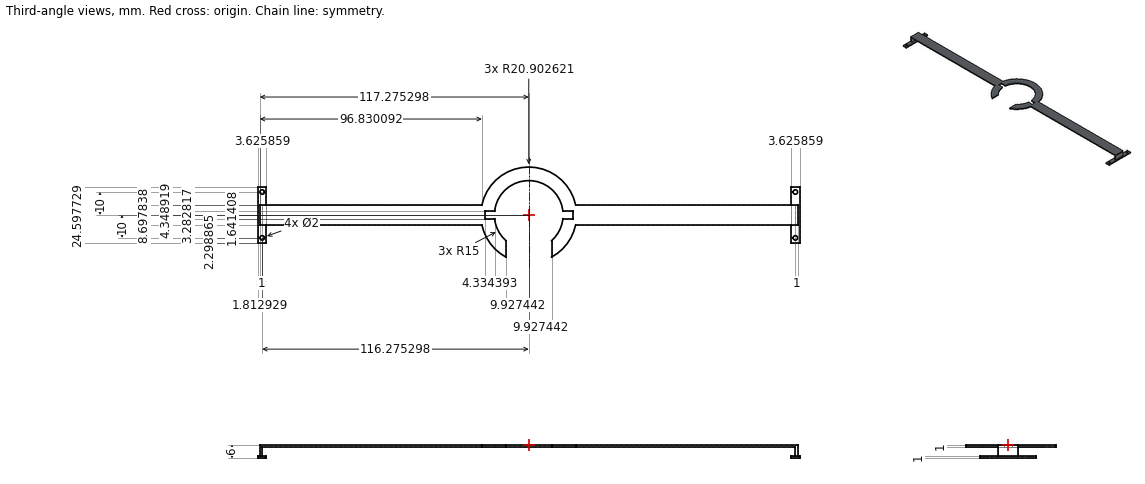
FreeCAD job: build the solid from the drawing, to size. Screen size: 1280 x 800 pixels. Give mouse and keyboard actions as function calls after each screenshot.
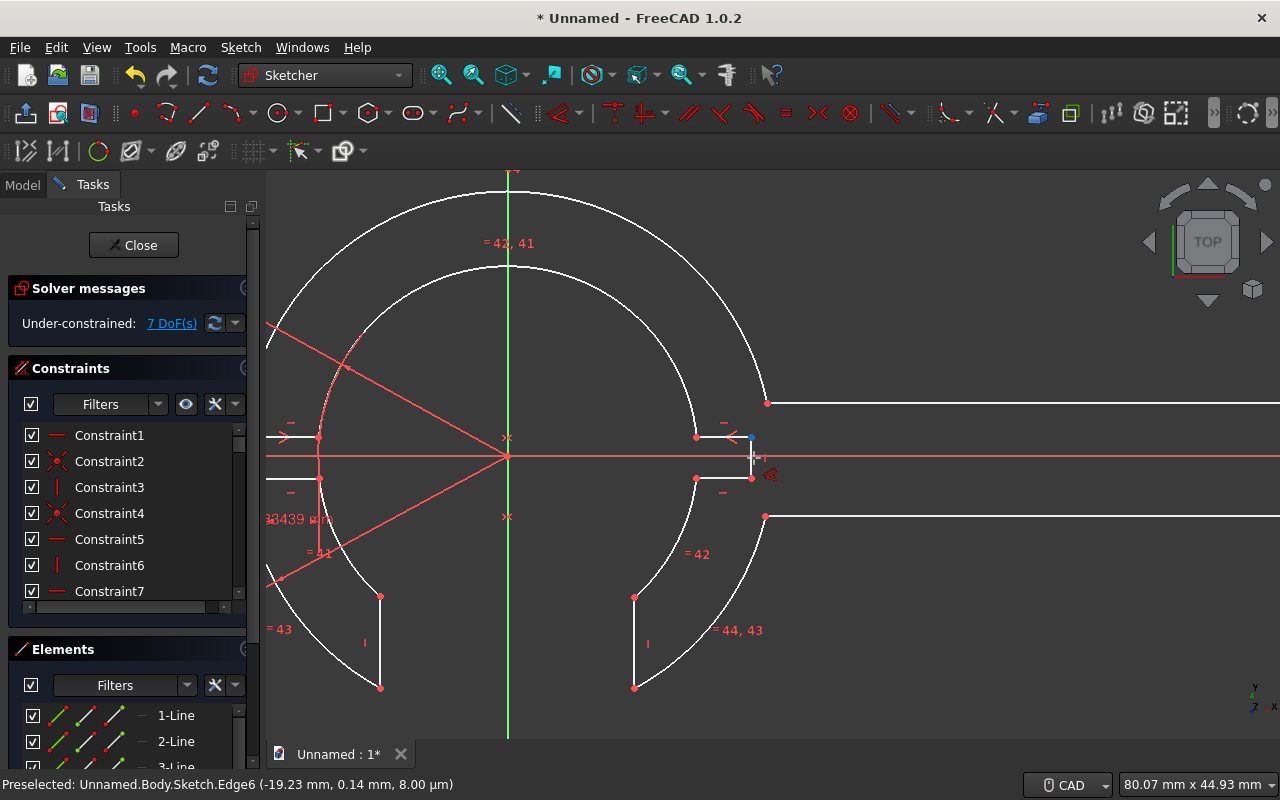
click(751, 454)
click(785, 472)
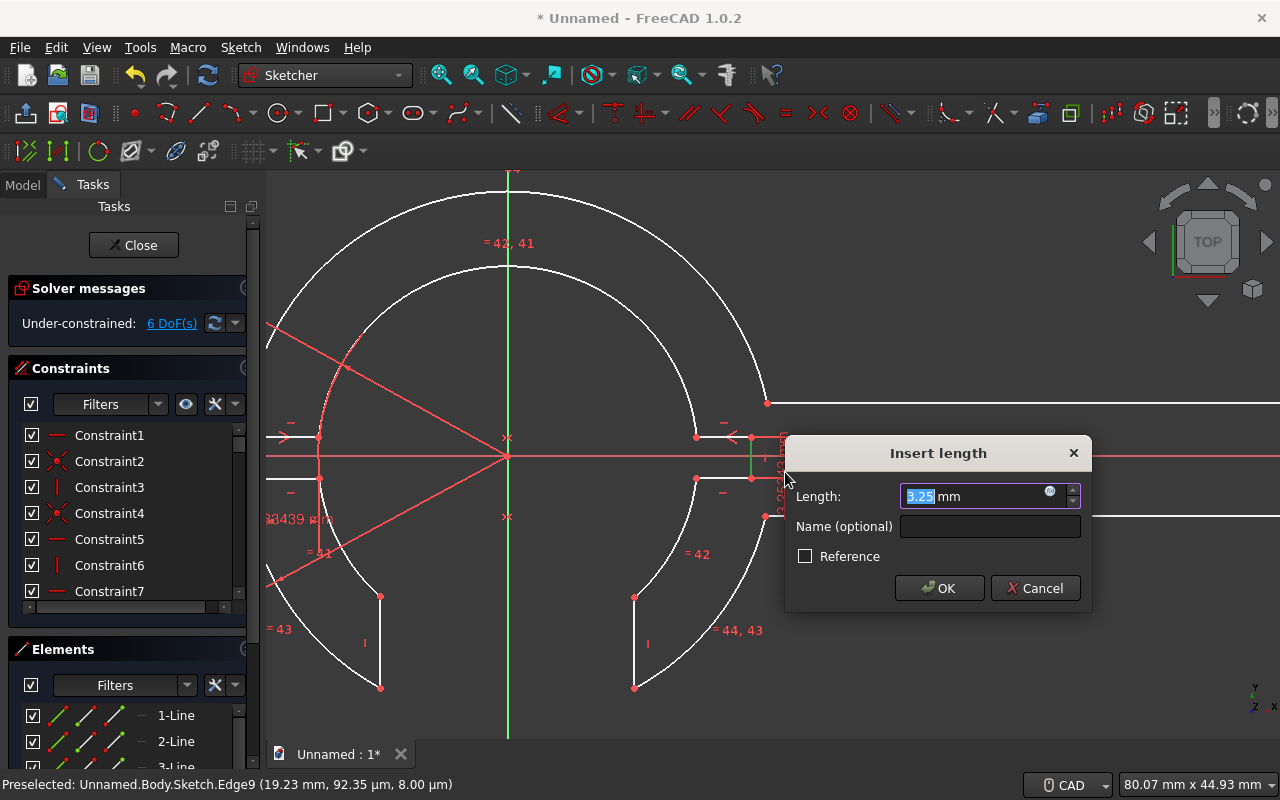
text(3.282817)
key(Return)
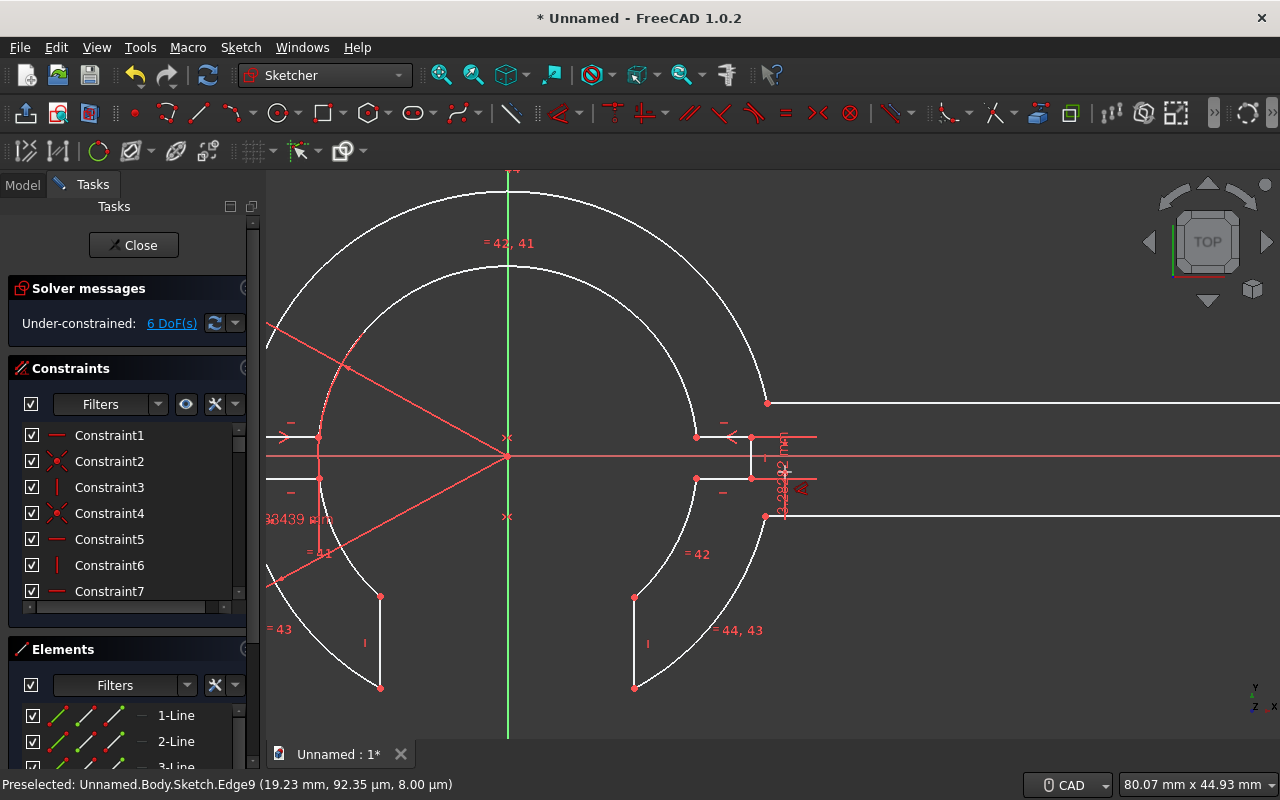
scroll(754, 458, down, 8)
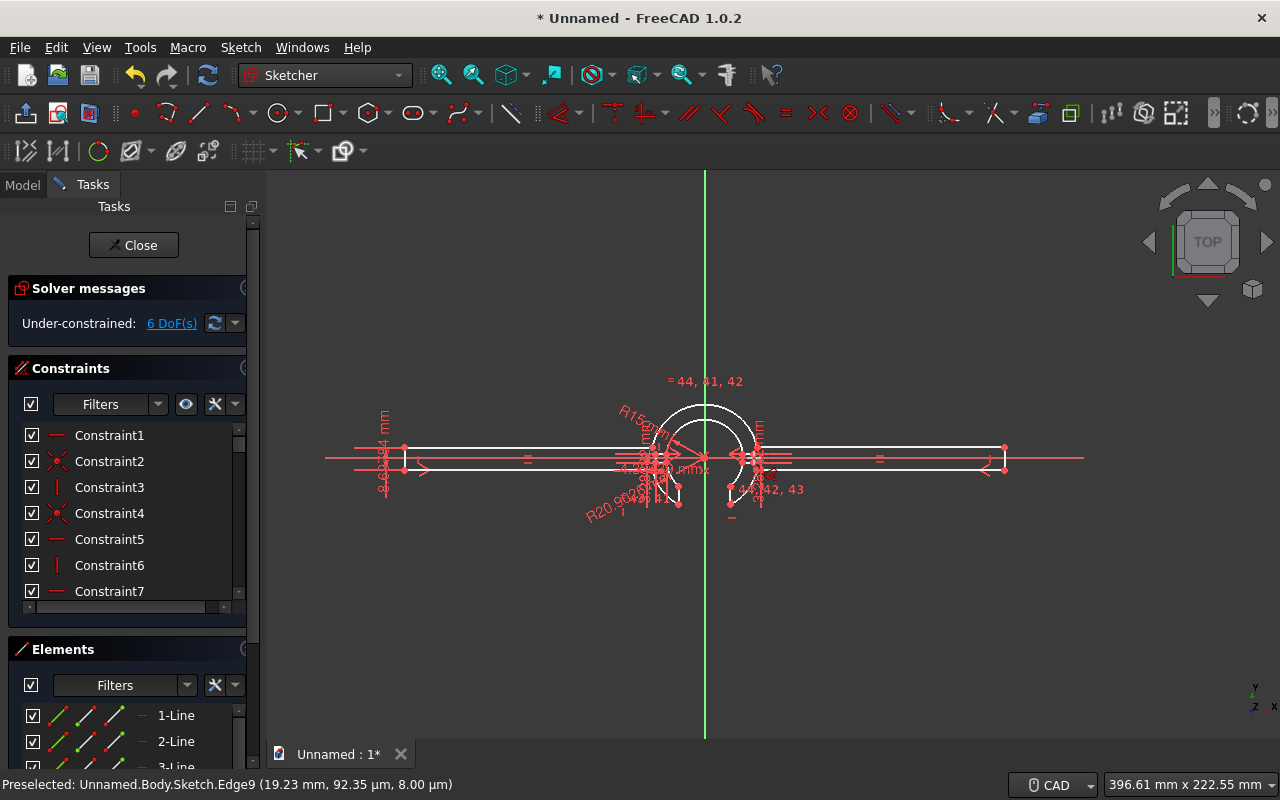
scroll(1005, 463, up, 5)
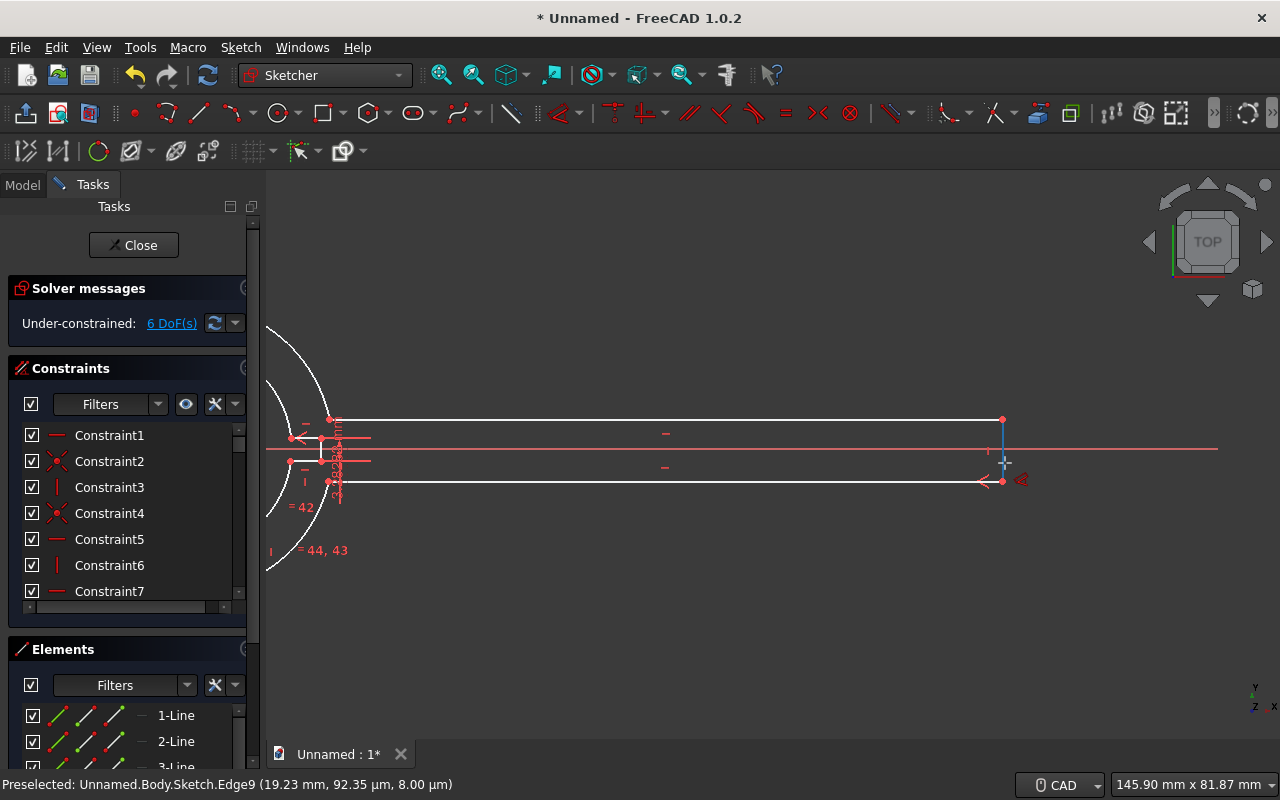
click(1003, 463)
click(1037, 465)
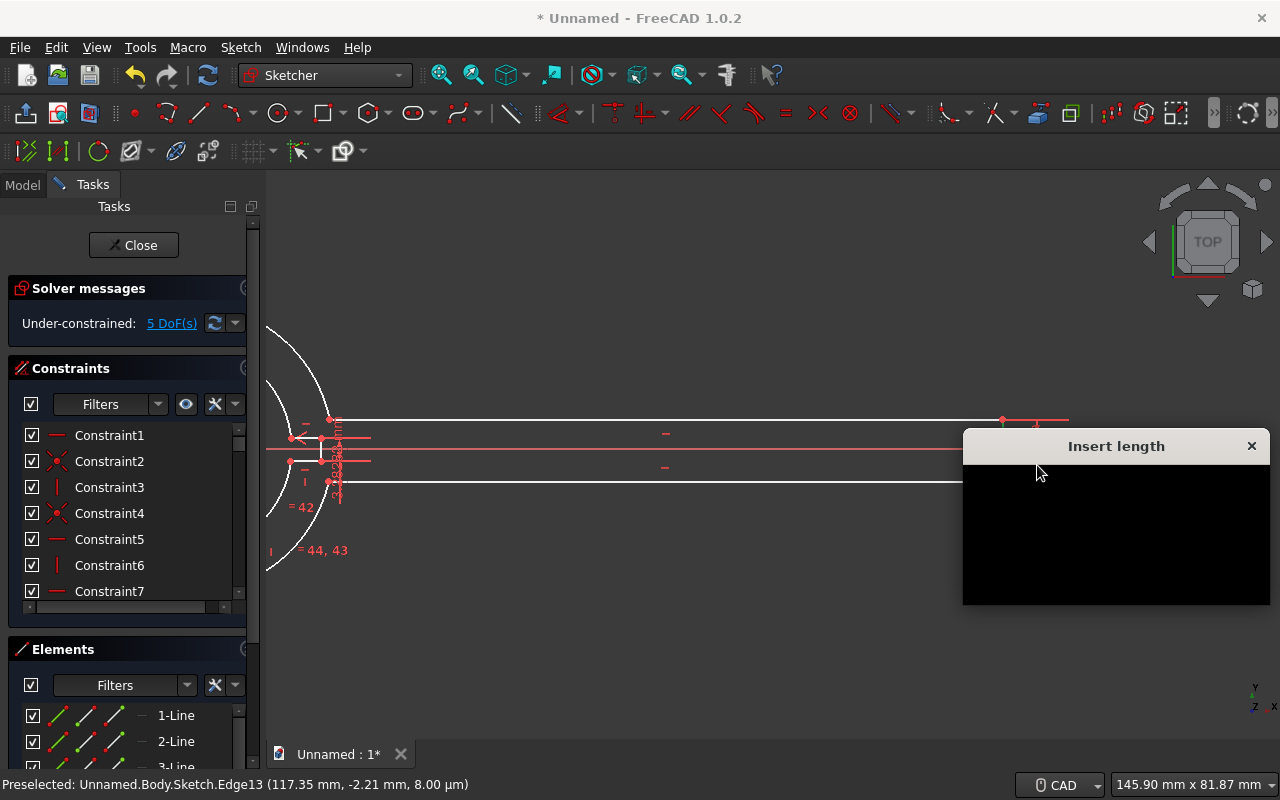
text(8.697838)
key(Return)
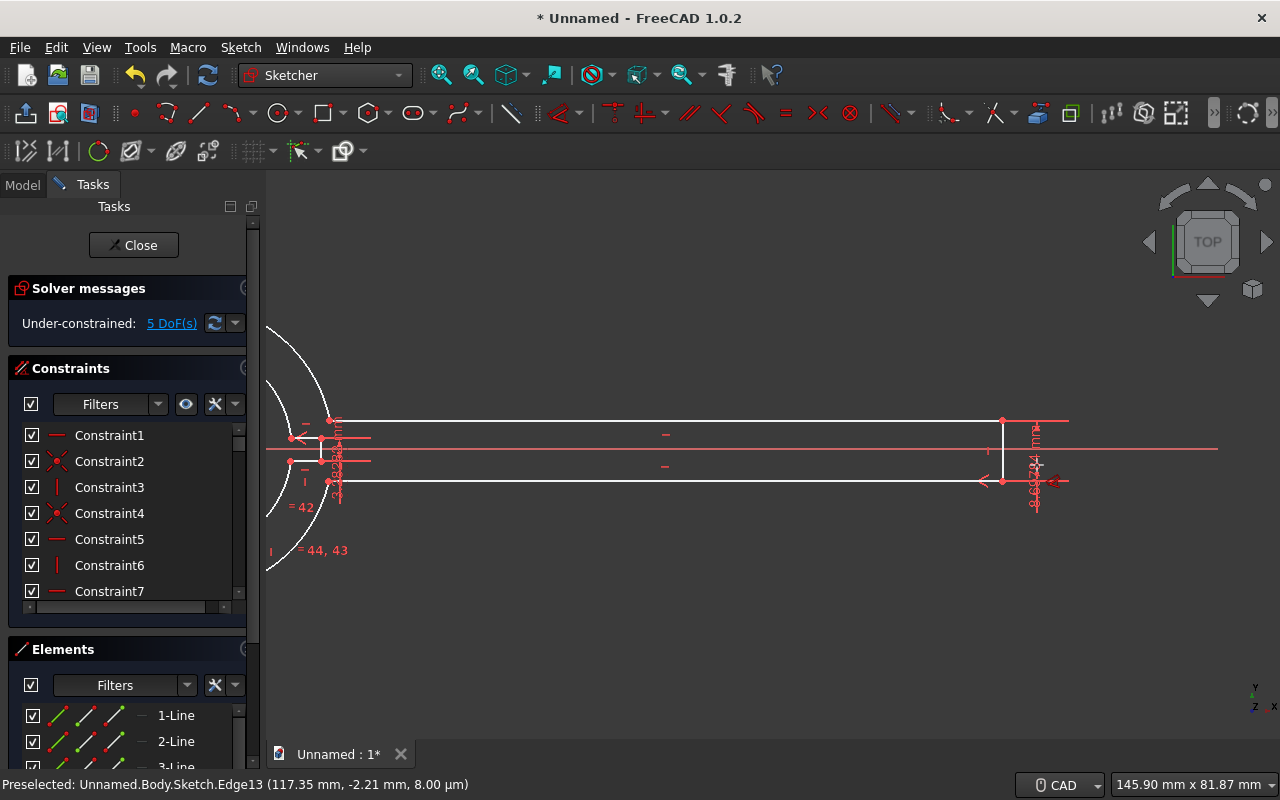
scroll(1005, 463, down, 5)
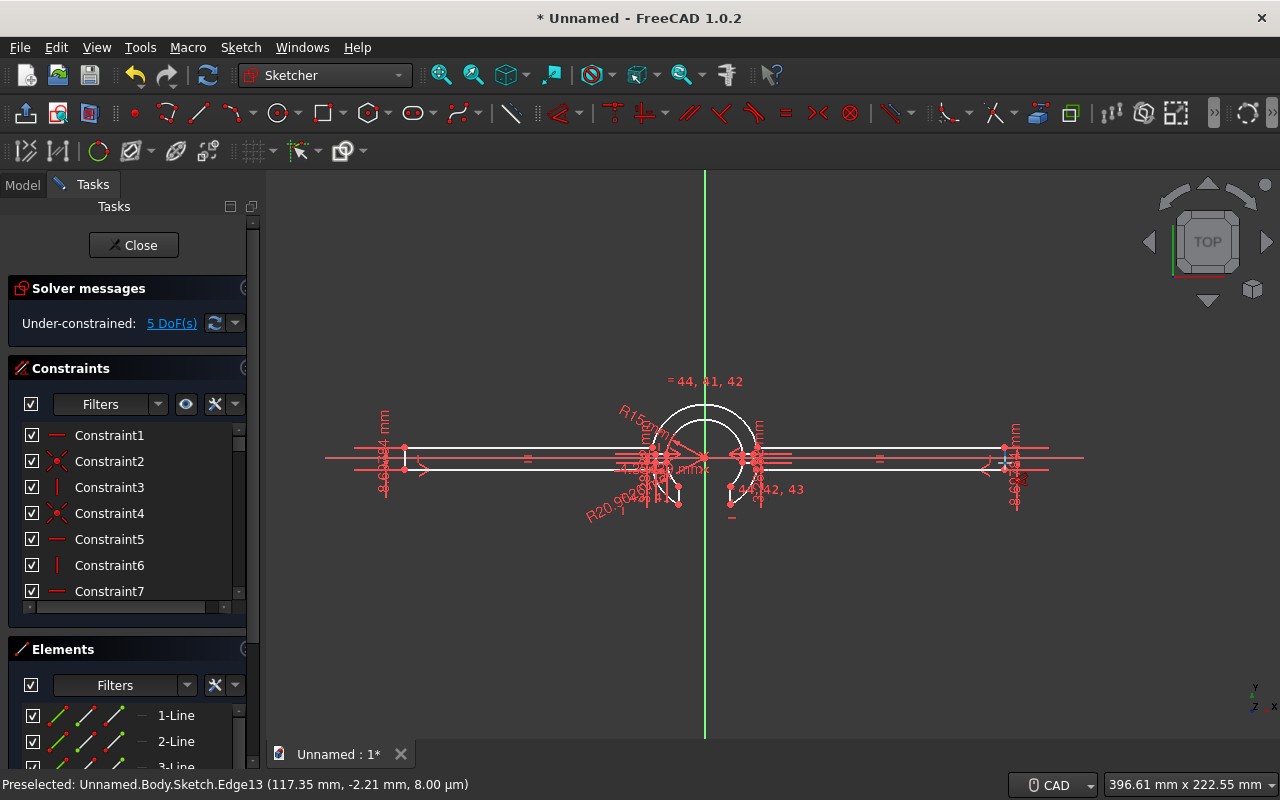
scroll(578, 448, up, 2)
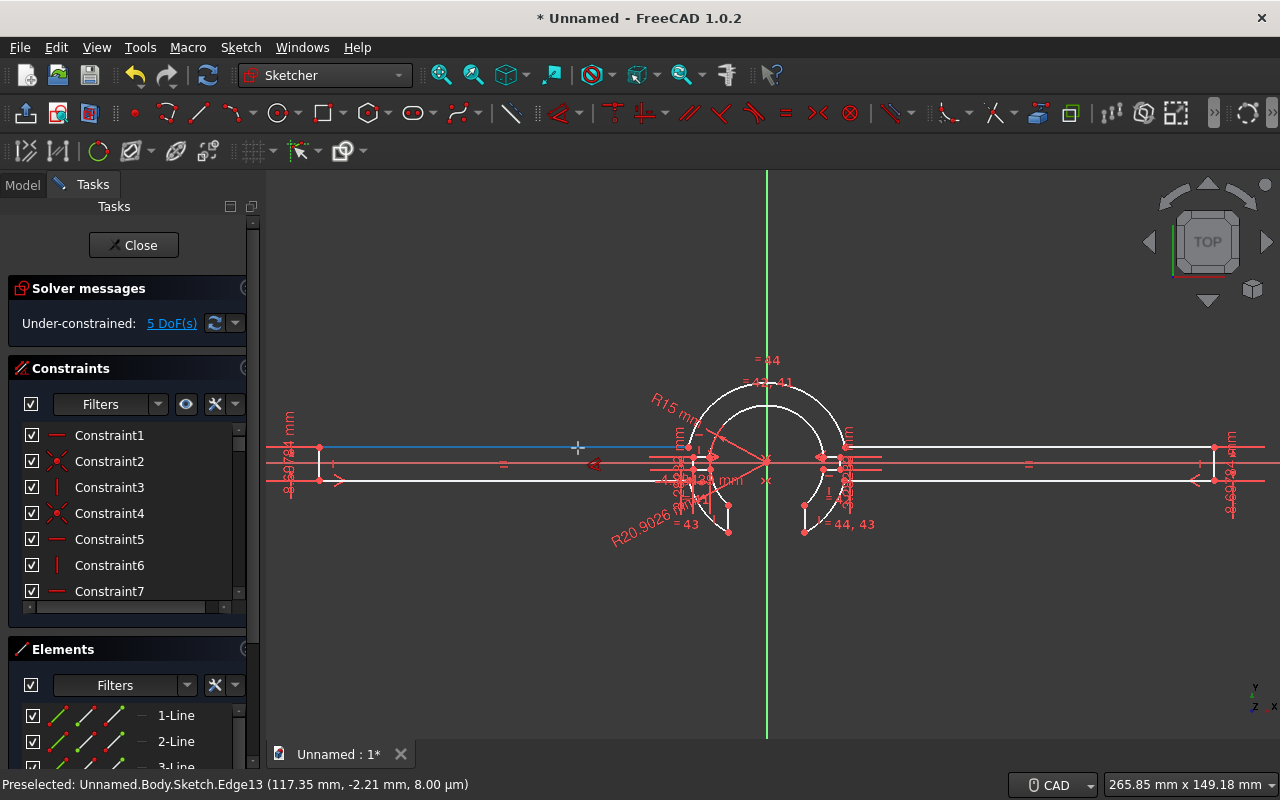
click(578, 447)
click(504, 413)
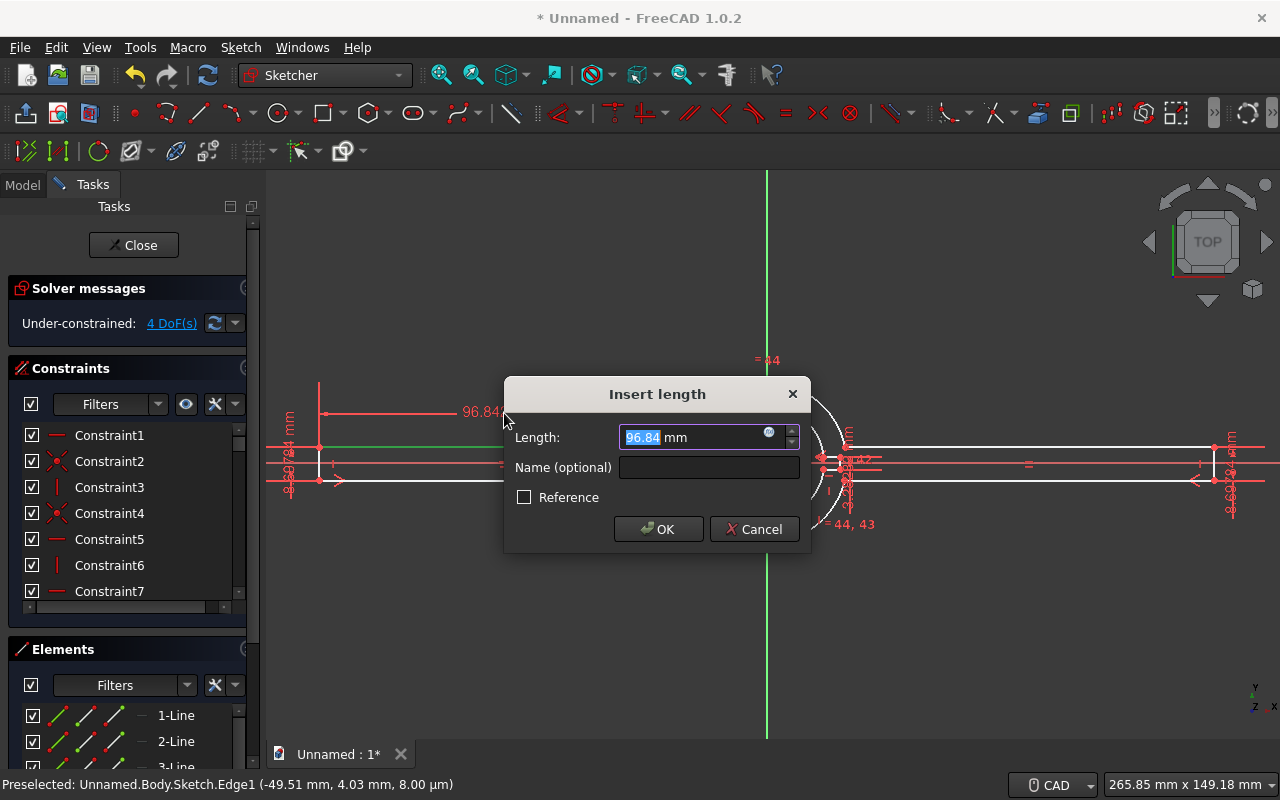
text(96.830092)
key(Return)